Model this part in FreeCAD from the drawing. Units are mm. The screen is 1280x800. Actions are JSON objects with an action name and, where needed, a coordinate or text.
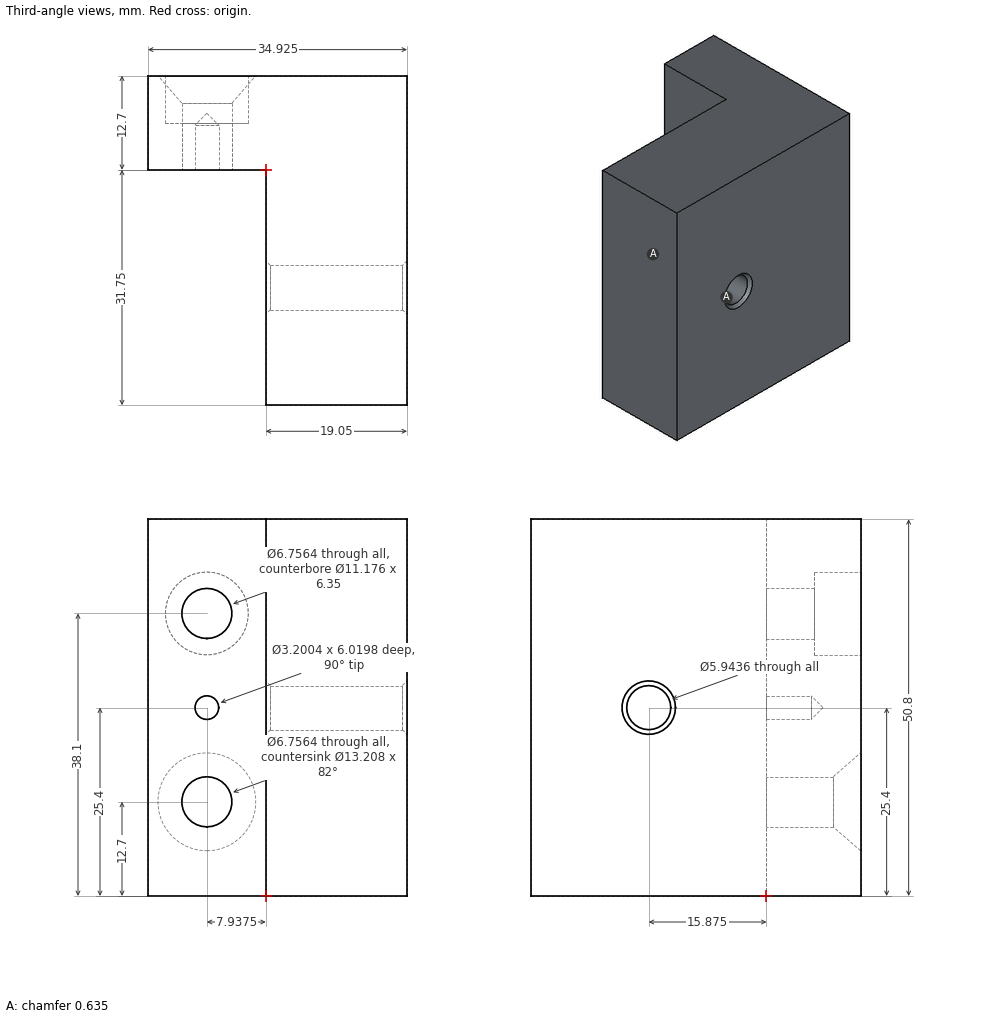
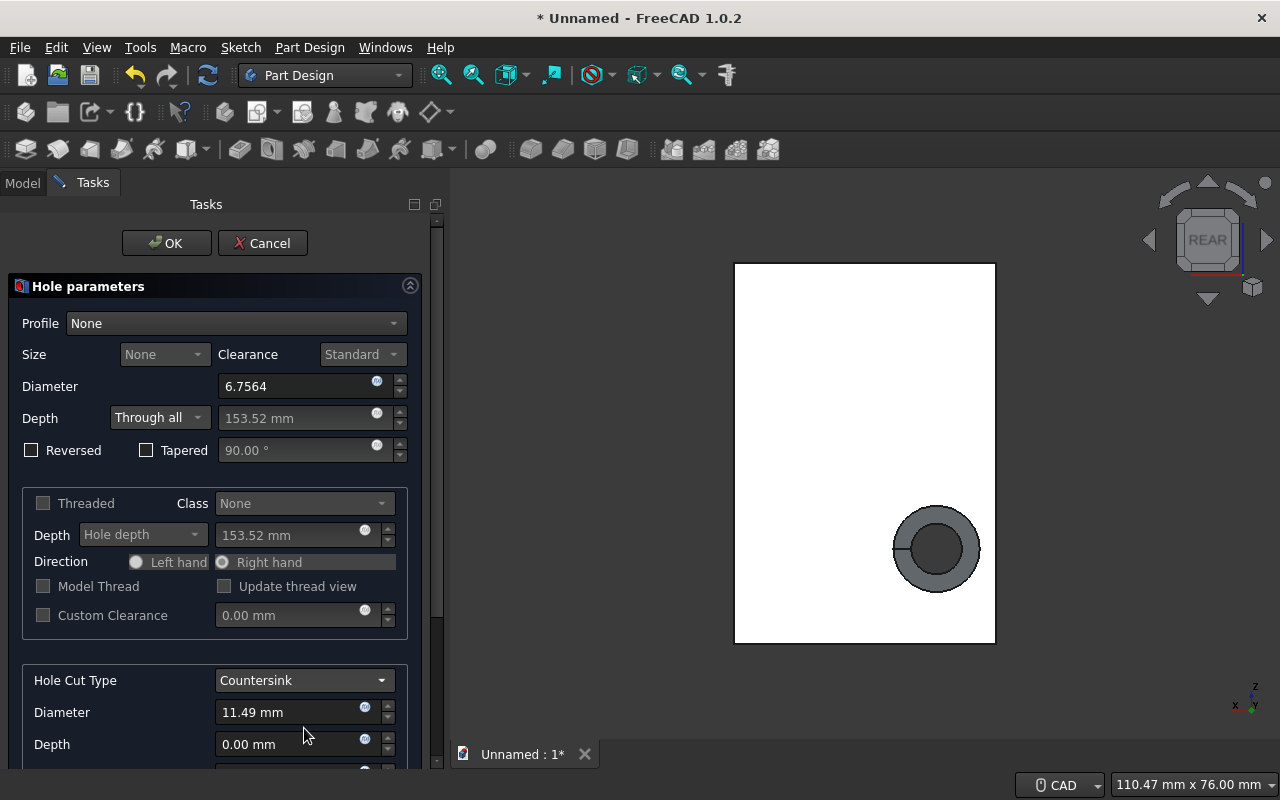
{"action": "scroll", "coordinate": [437, 491], "scroll_direction": "down", "scroll_amount": 2}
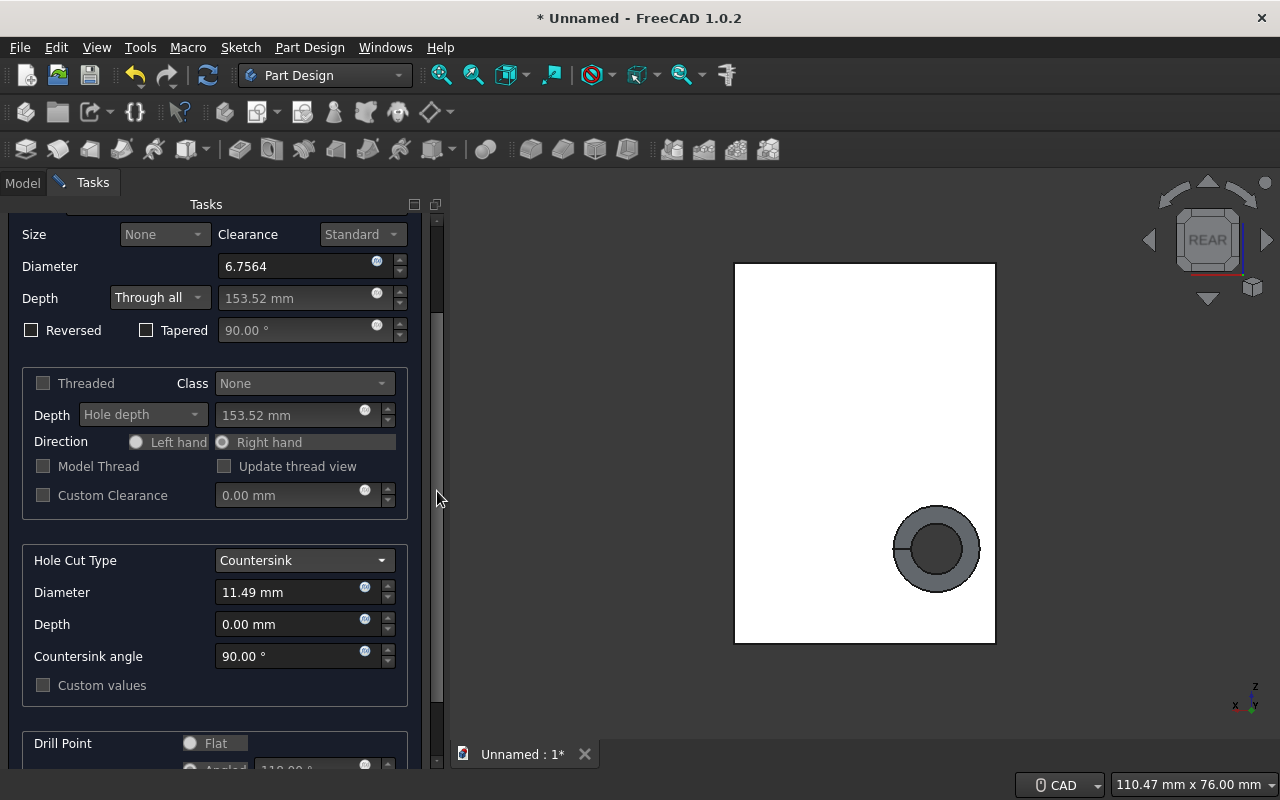
{"action": "triple_click", "coordinate": [298, 656]}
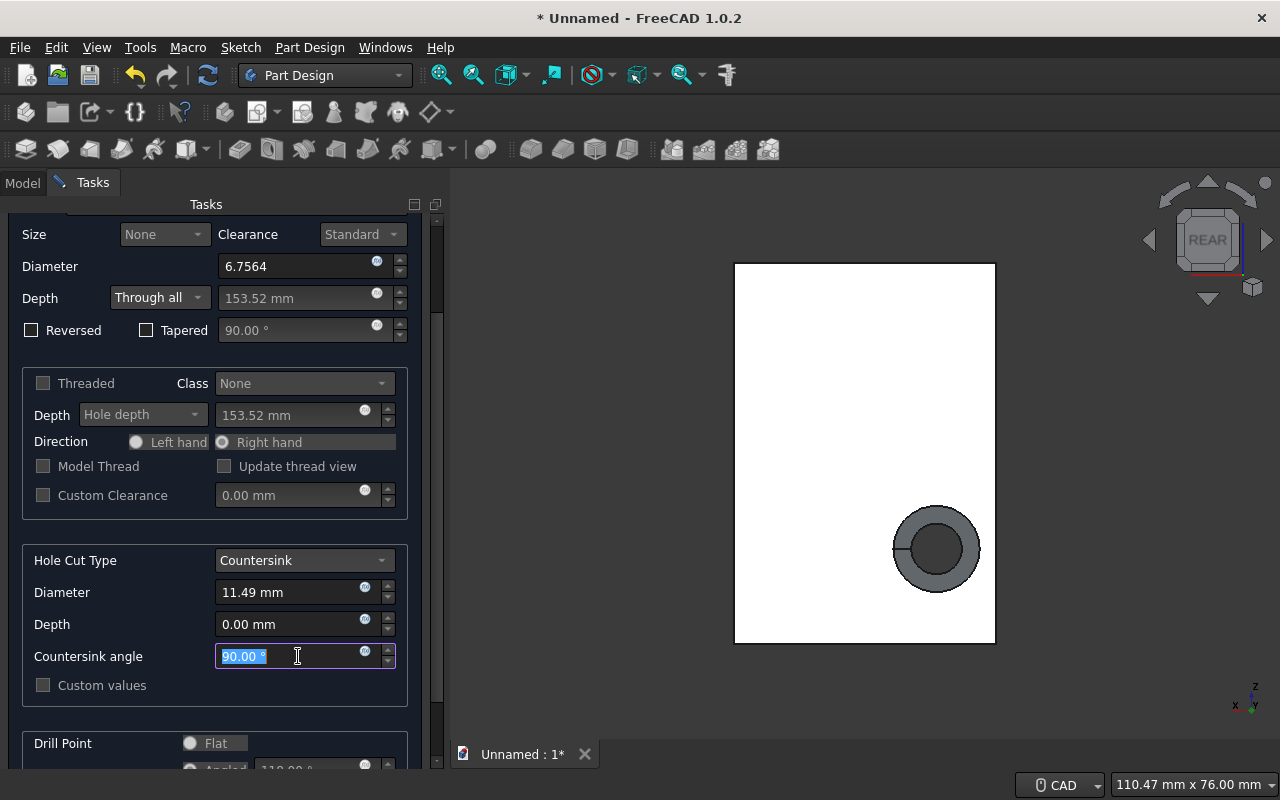
{"action": "type", "text": "82"}
{"action": "key", "text": "Tab"}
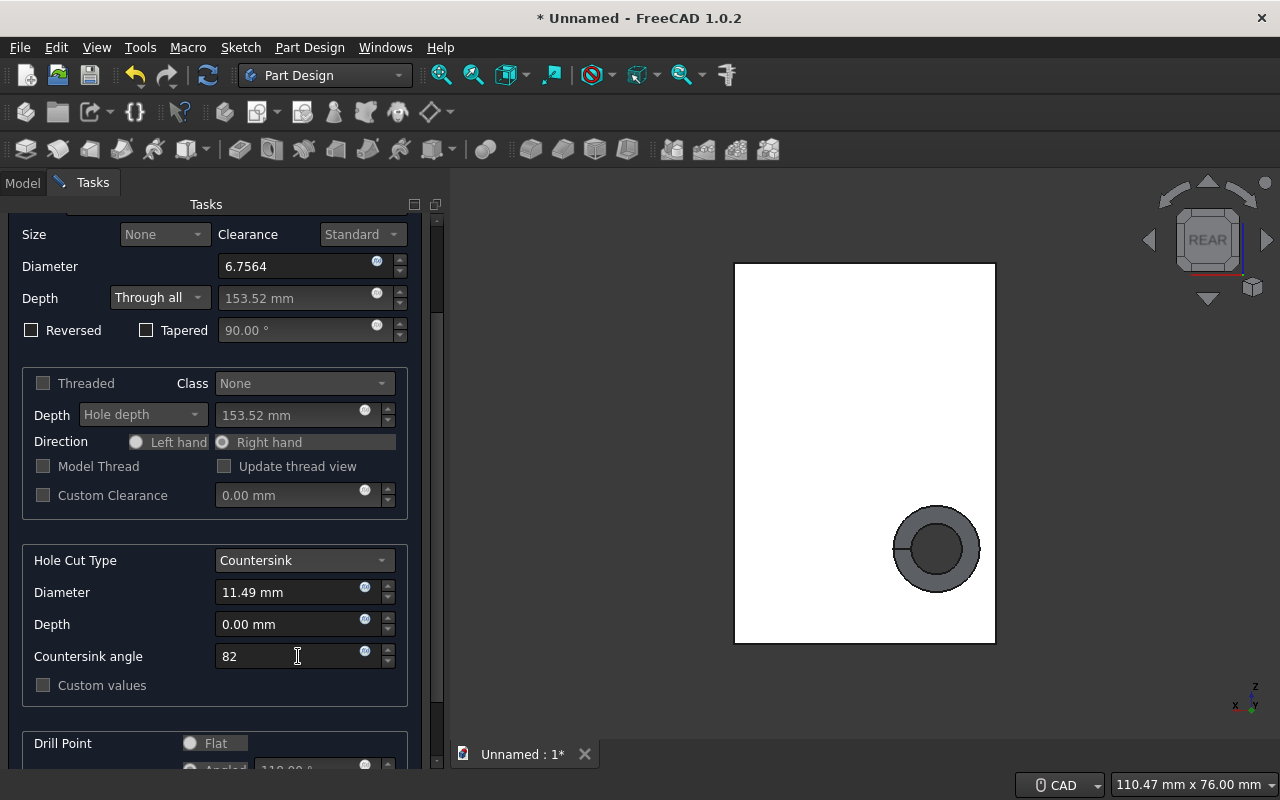
{"action": "triple_click", "coordinate": [298, 592]}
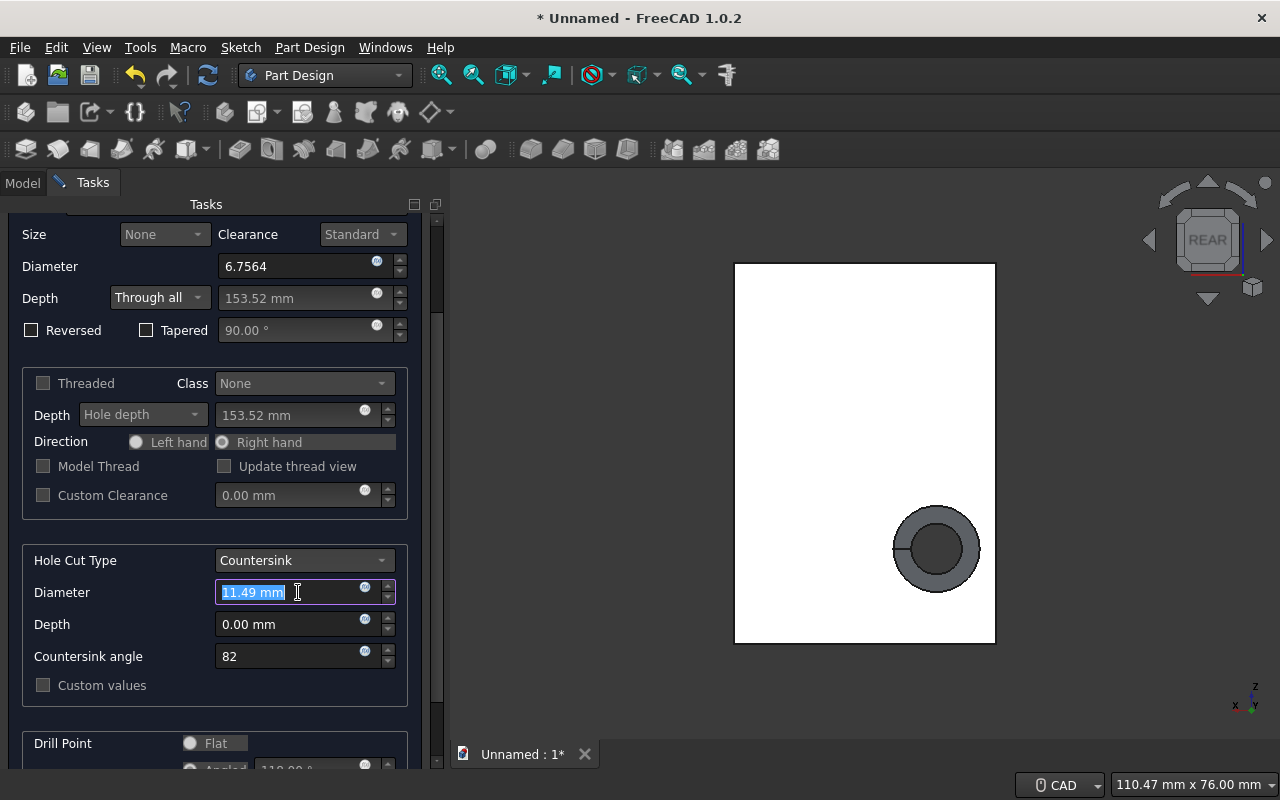
{"action": "type", "text": "13.208"}
{"action": "key", "text": "Tab"}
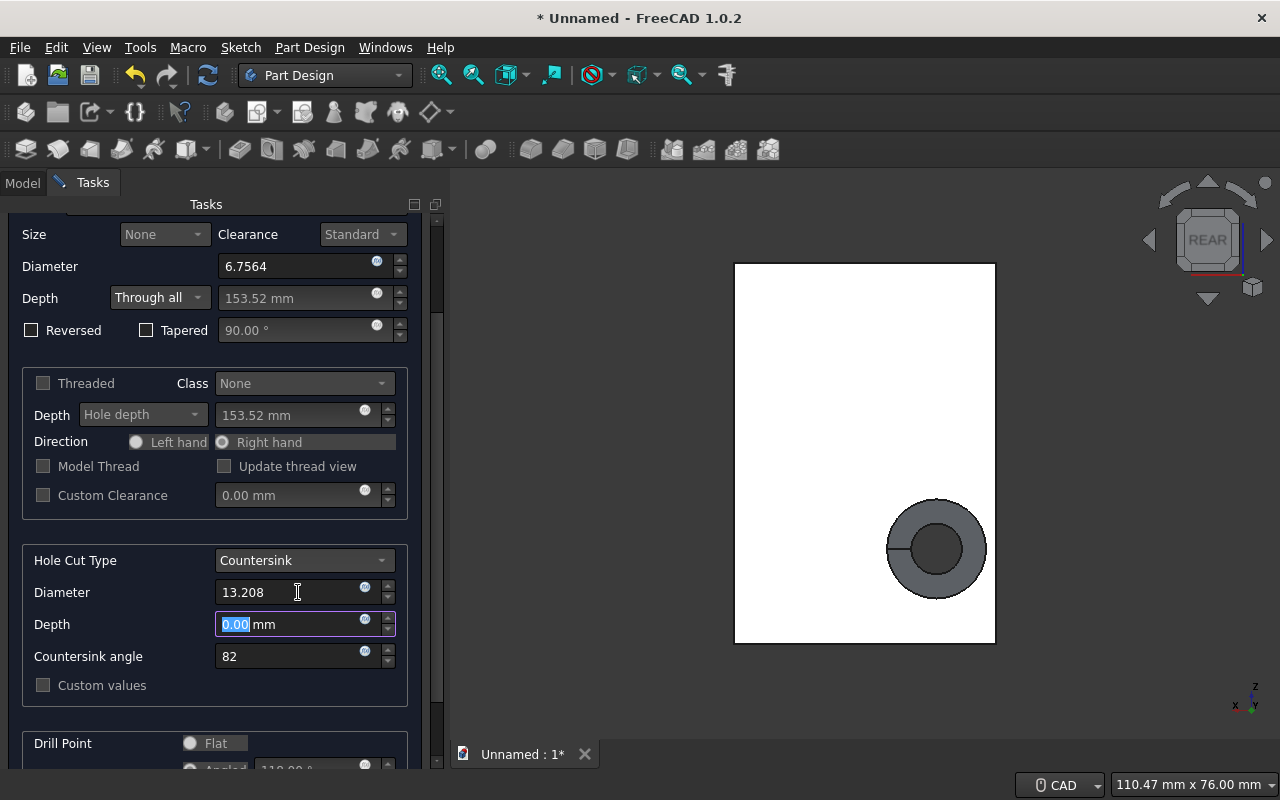
{"action": "scroll", "coordinate": [437, 491], "scroll_direction": "up", "scroll_amount": 3}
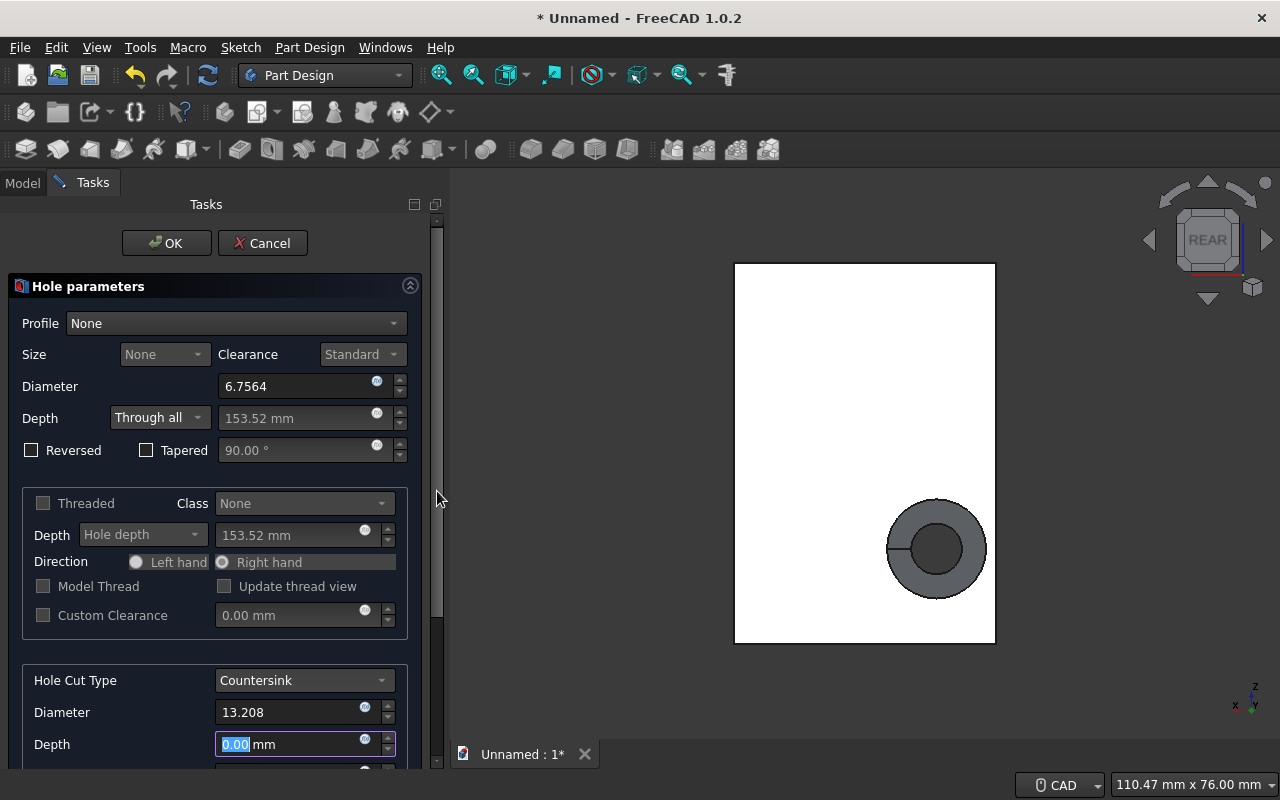
{"action": "left_click", "coordinate": [167, 243]}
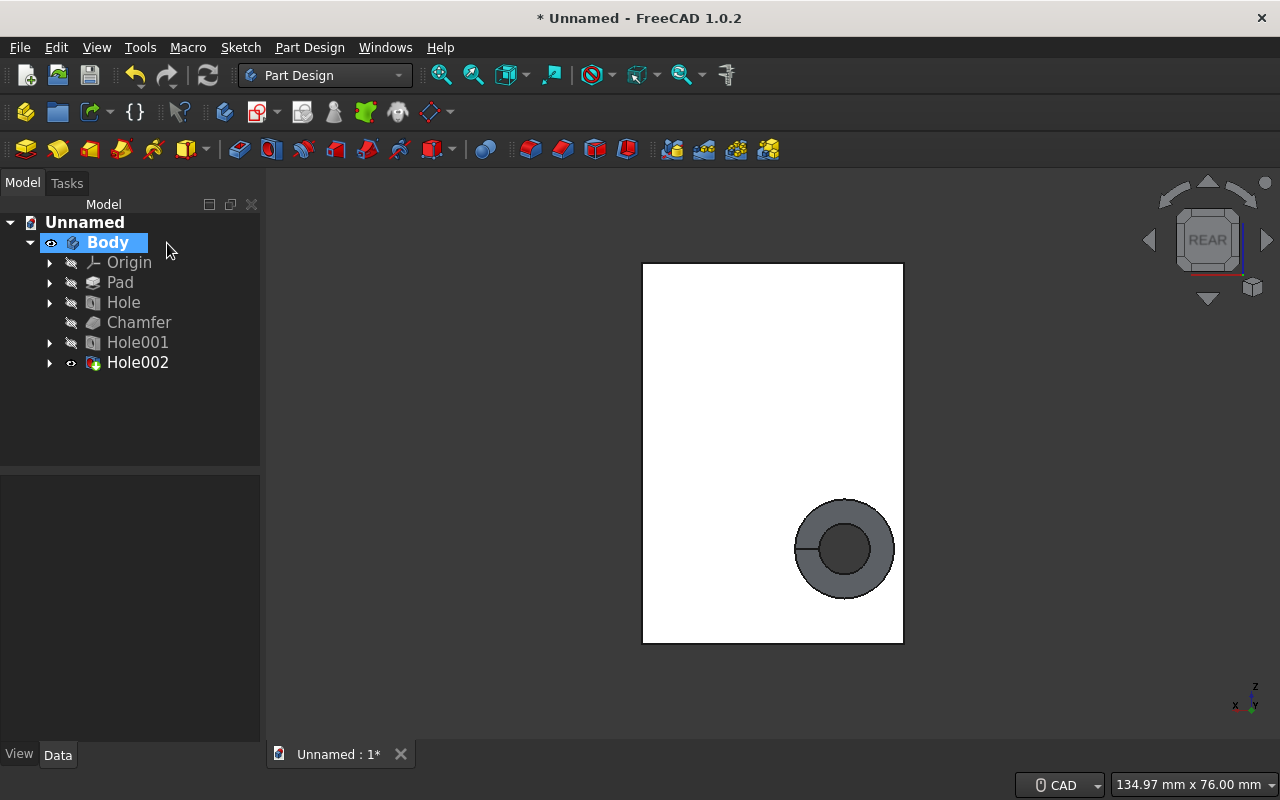
{"action": "left_click", "coordinate": [773, 398]}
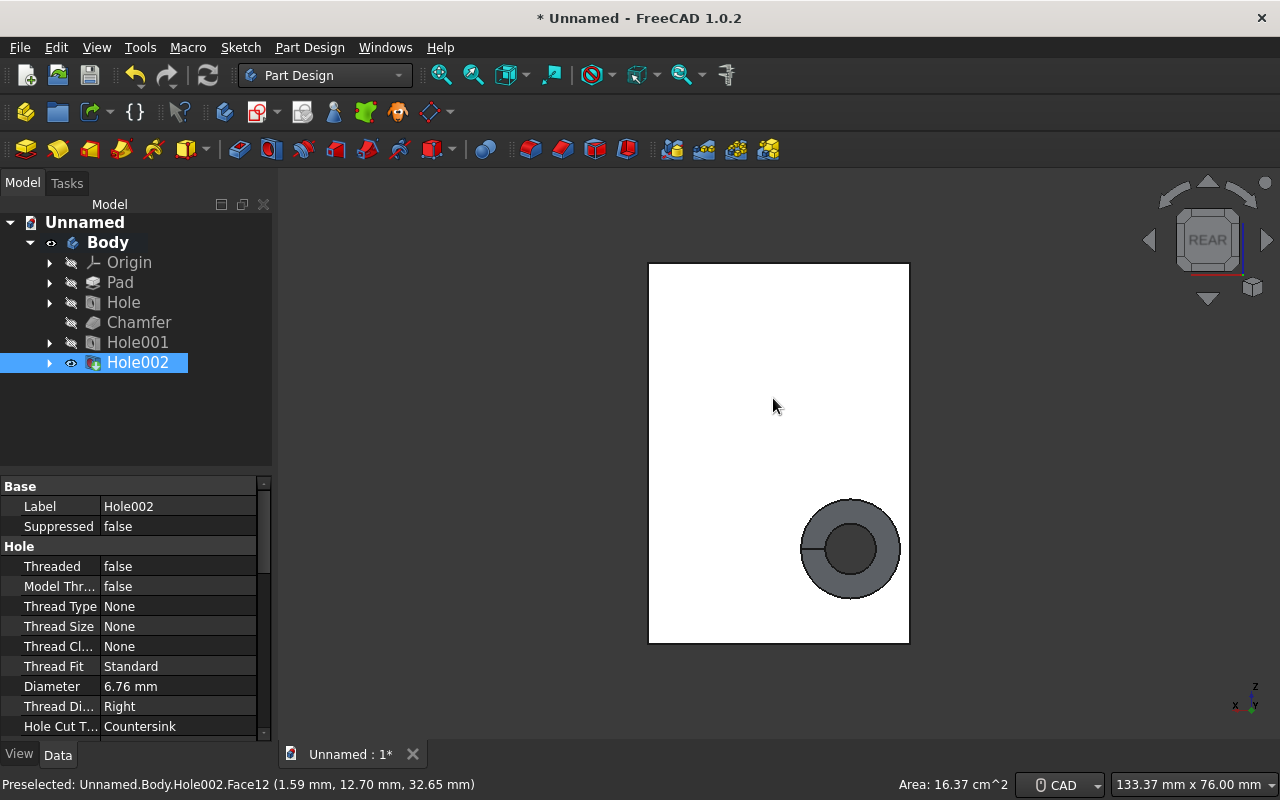
{"action": "left_click", "coordinate": [258, 112]}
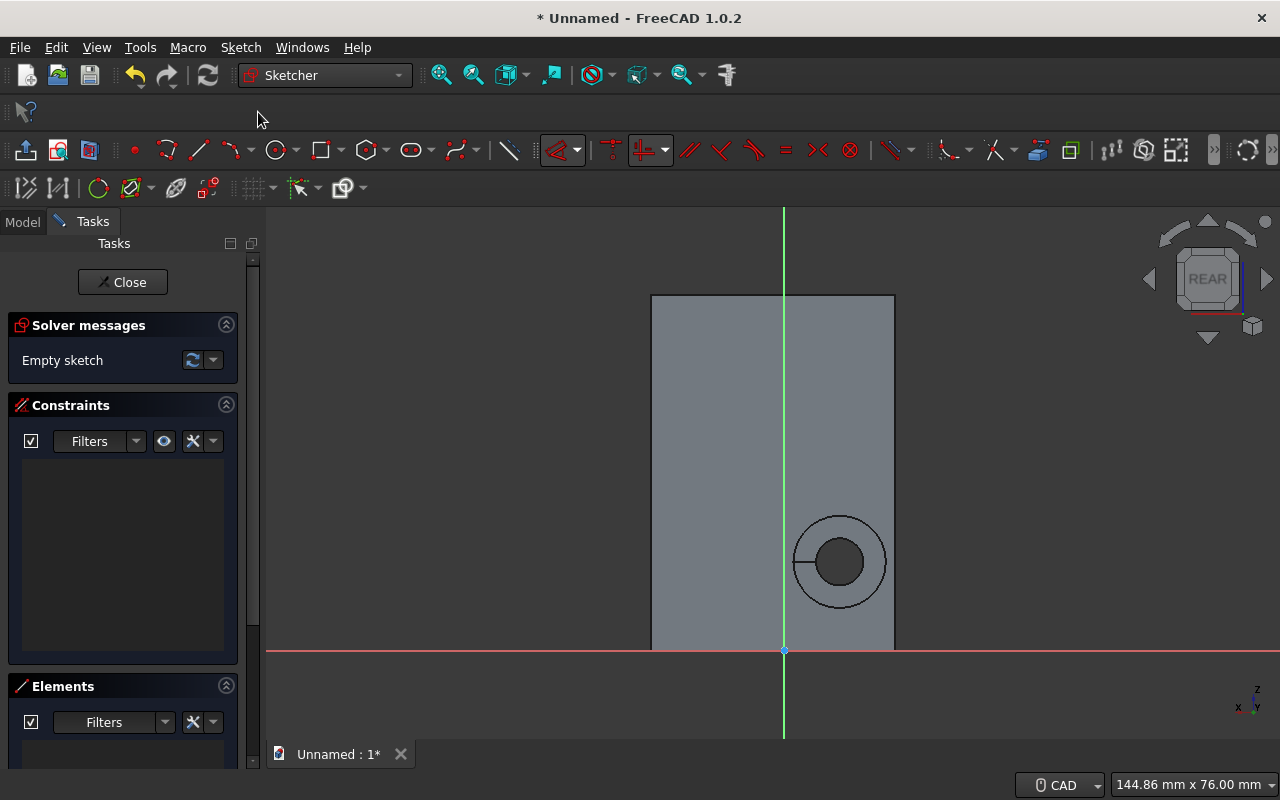
{"action": "scroll", "coordinate": [861, 370], "scroll_direction": "up", "scroll_amount": 10}